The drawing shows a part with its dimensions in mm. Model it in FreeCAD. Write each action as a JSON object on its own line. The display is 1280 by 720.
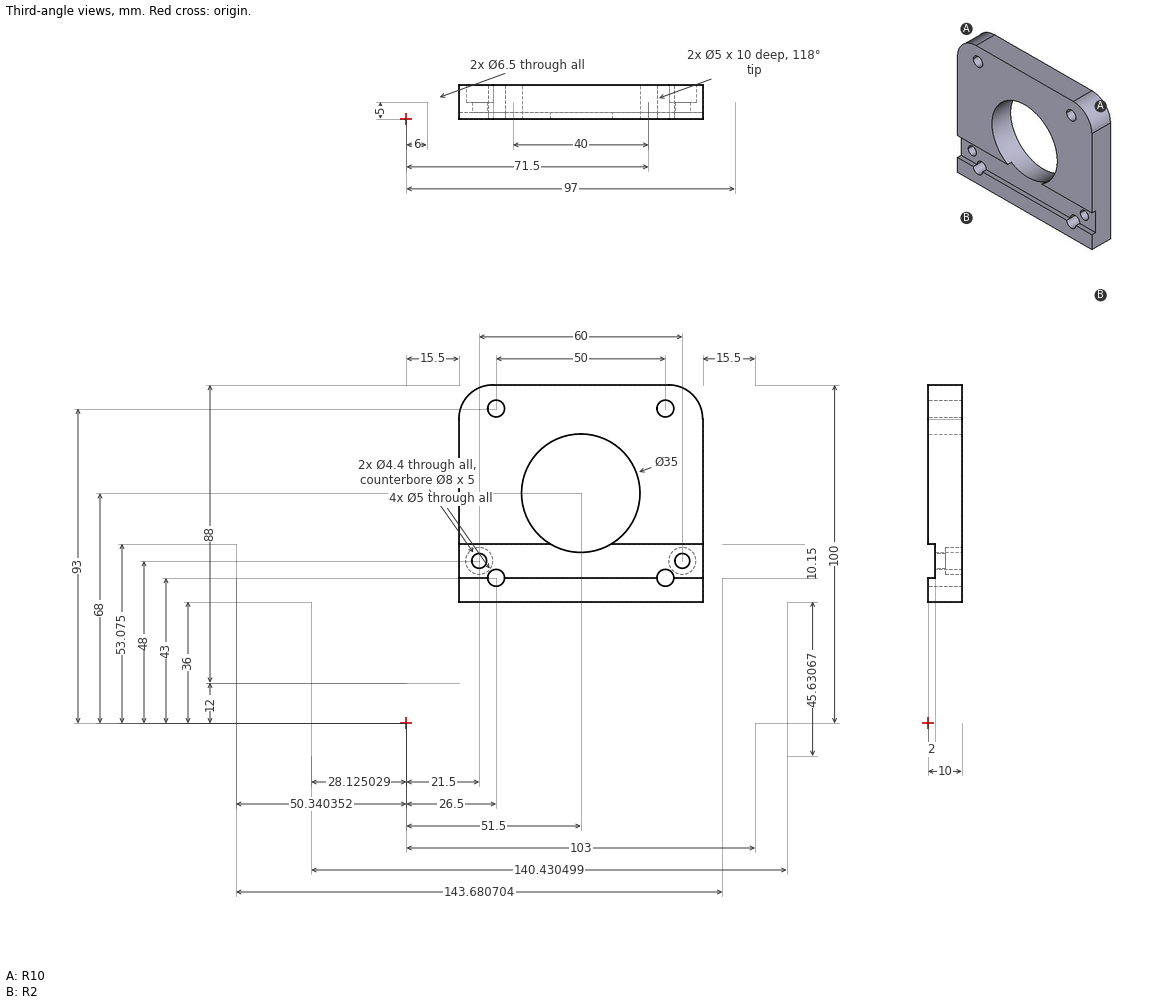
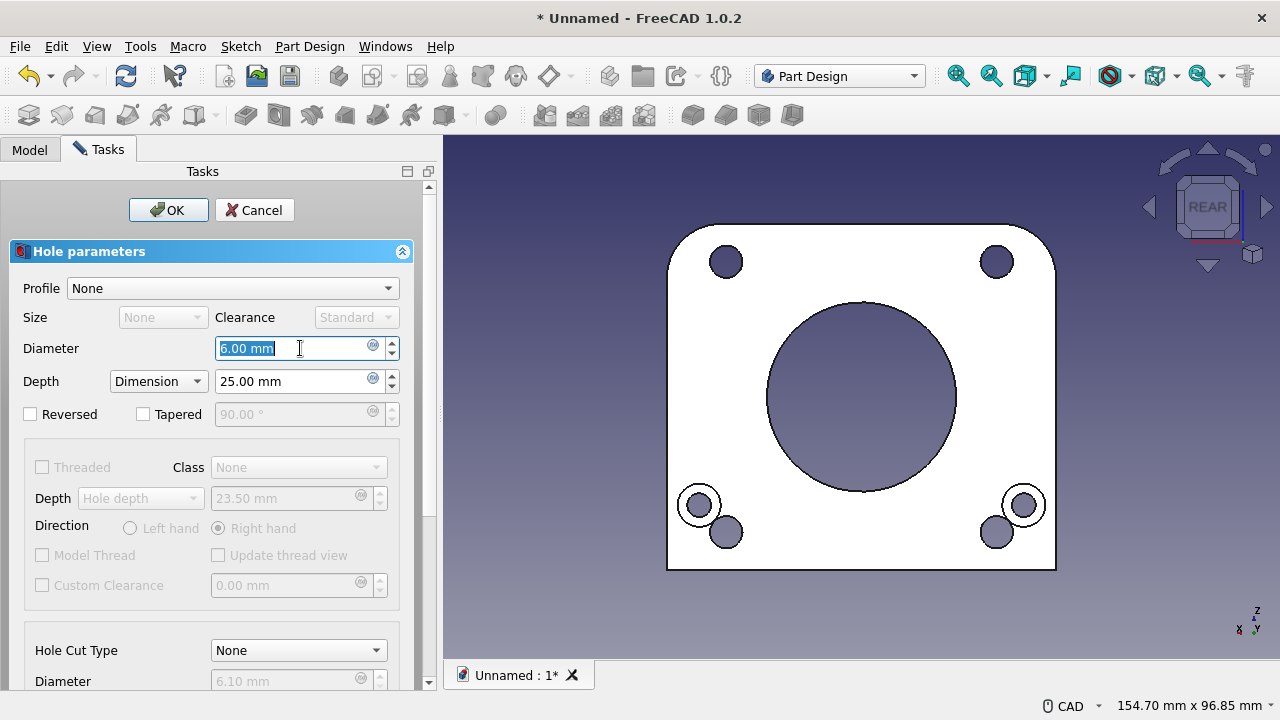
{"action": "type", "text": "5"}
{"action": "key", "text": "Tab"}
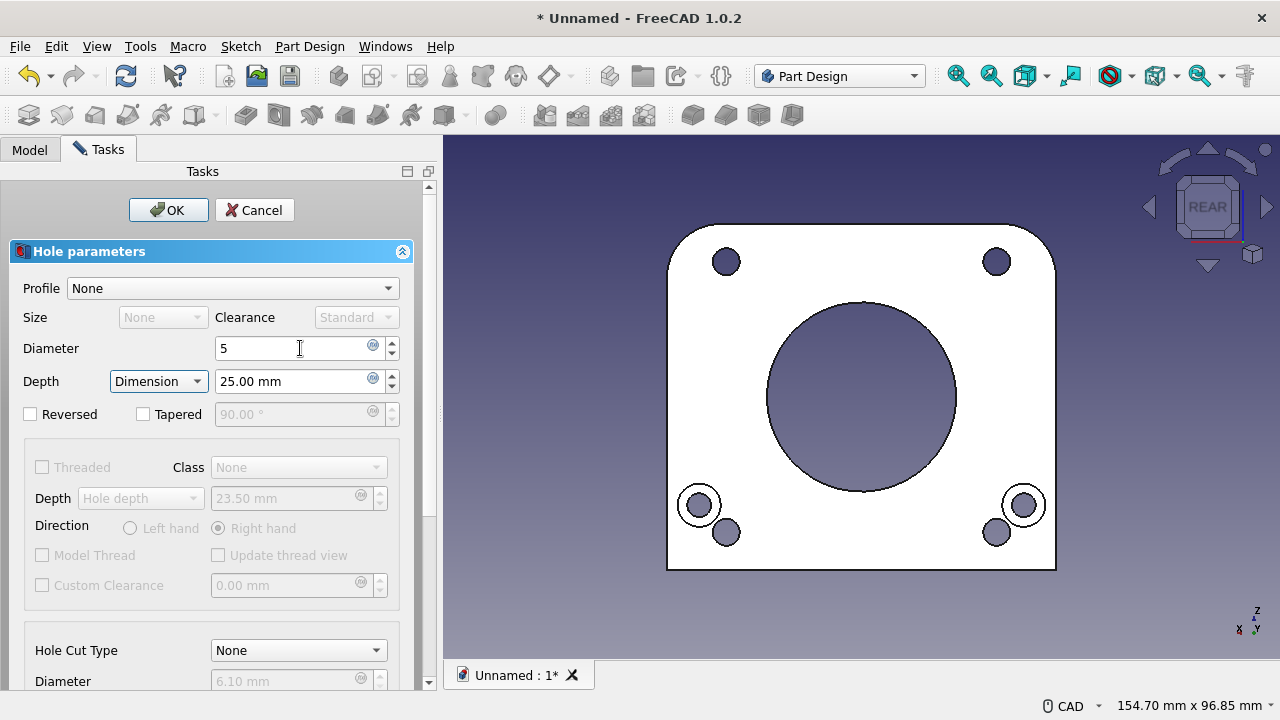
{"action": "left_click", "coordinate": [160, 382]}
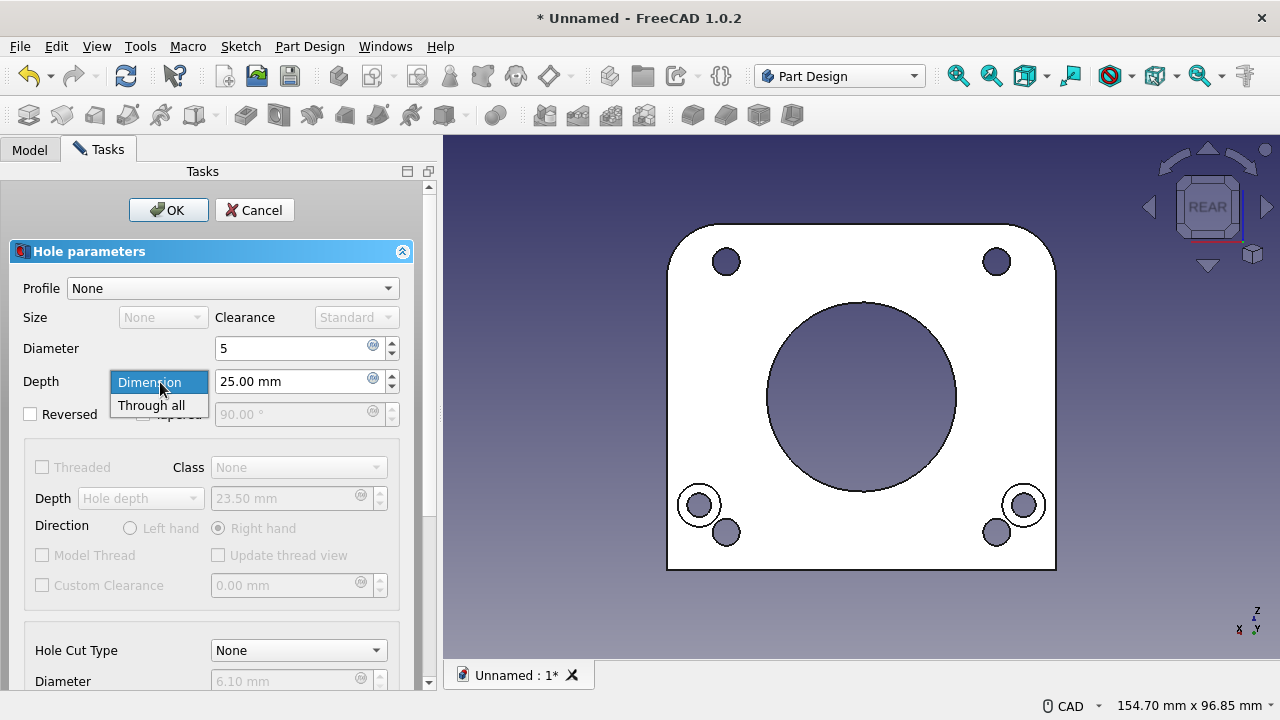
{"action": "left_click", "coordinate": [158, 406]}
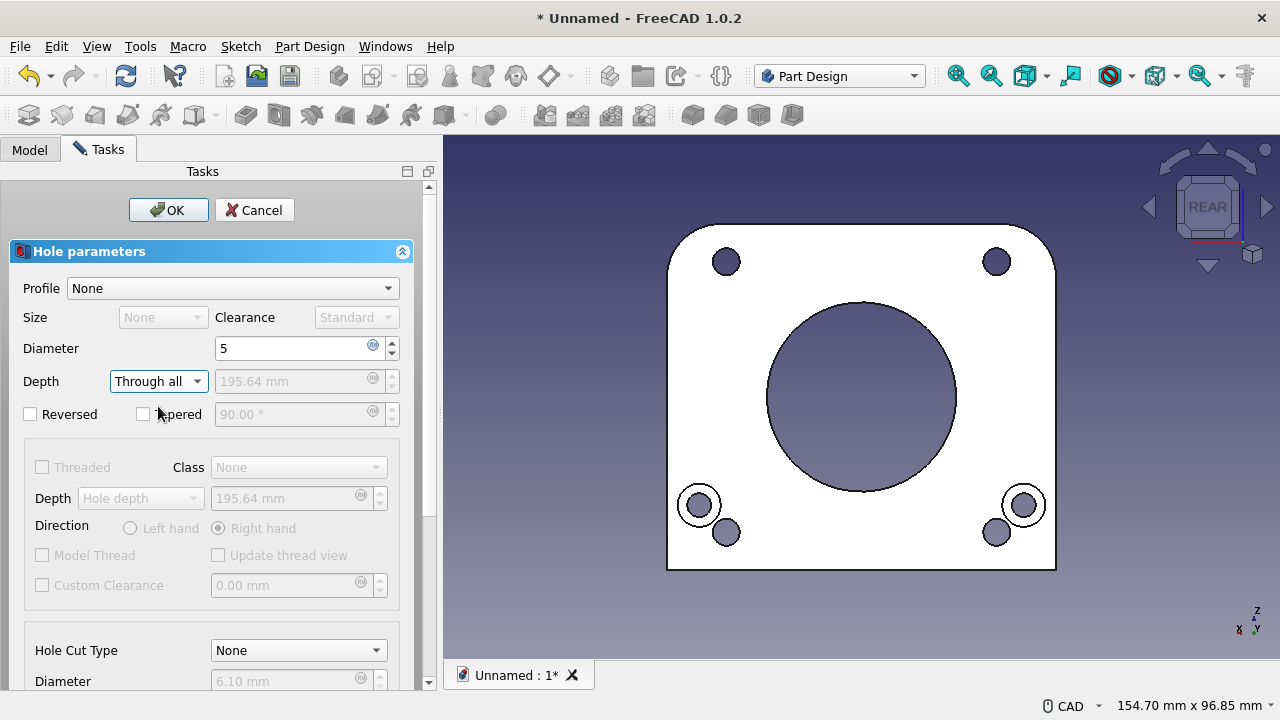
{"action": "left_click", "coordinate": [169, 210]}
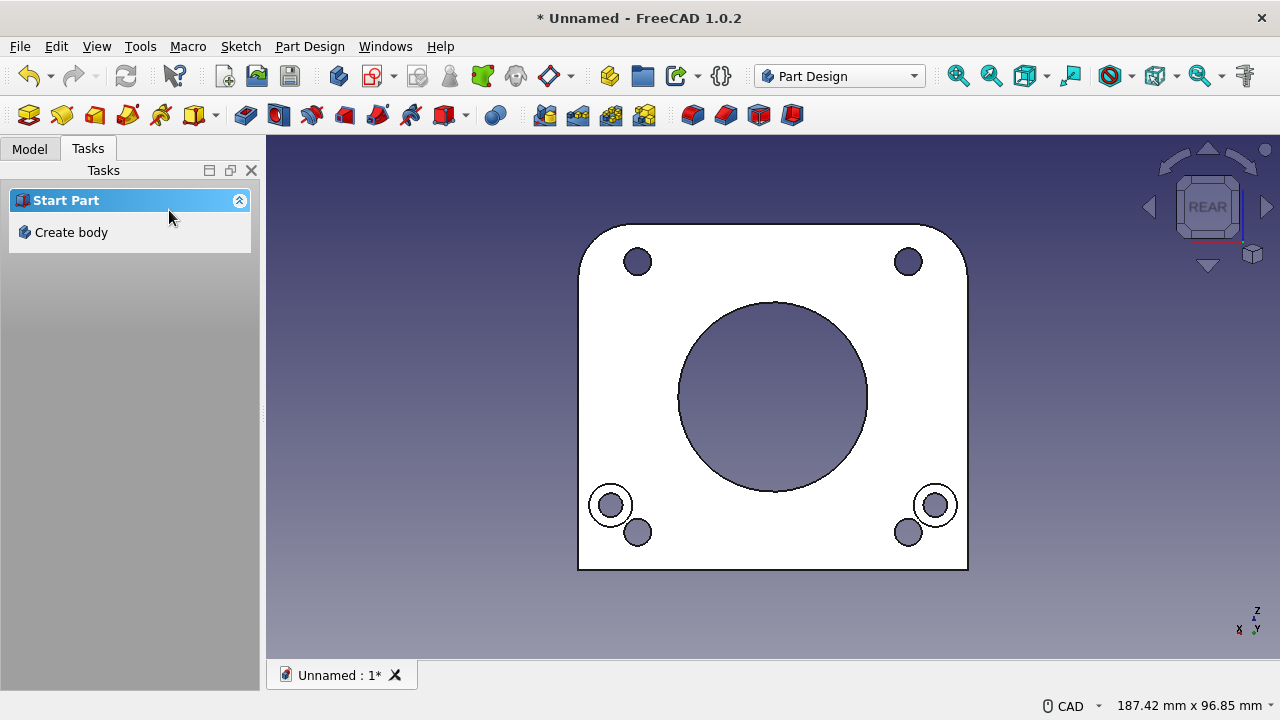
{"action": "key", "text": "0"}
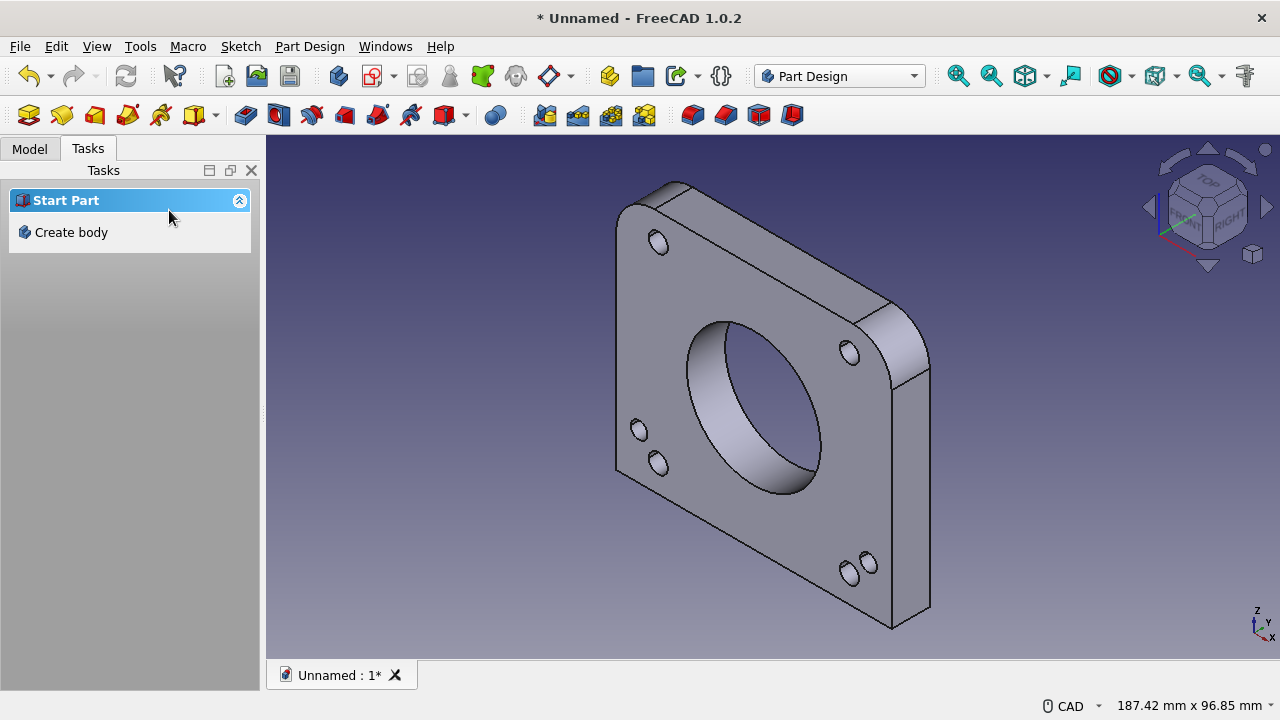
{"action": "left_click", "coordinate": [675, 442]}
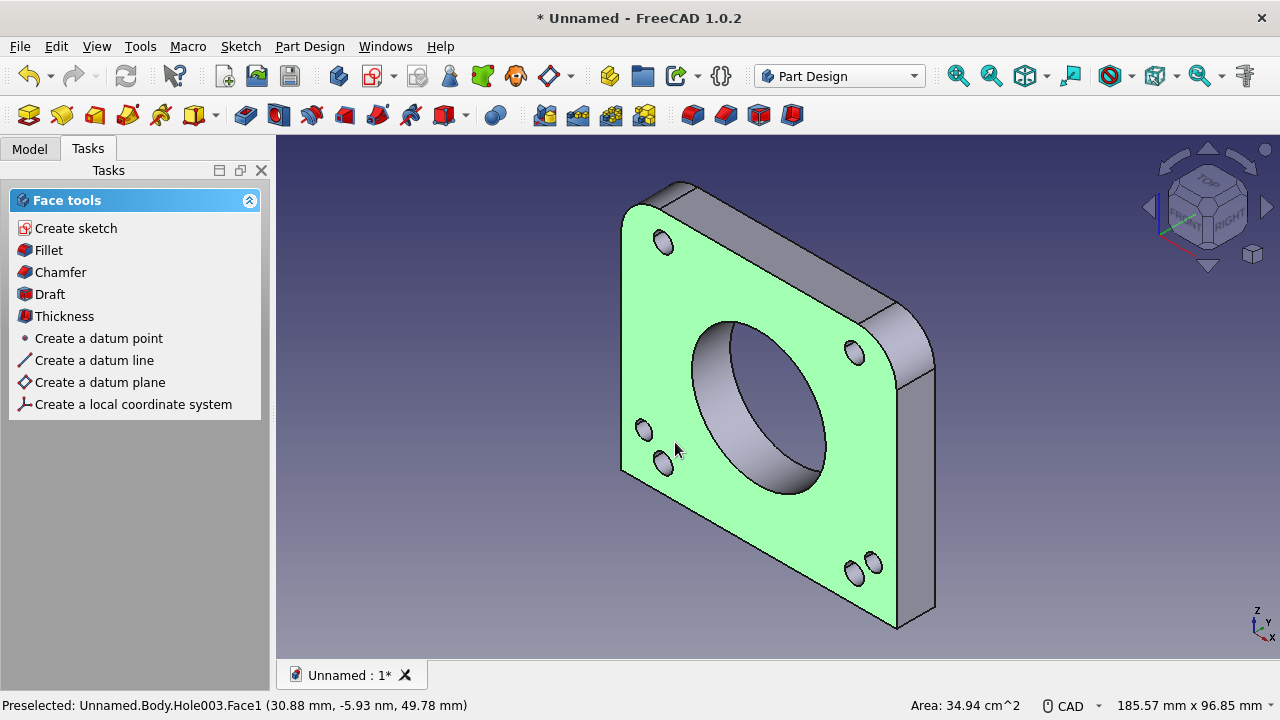
{"action": "left_click", "coordinate": [372, 76]}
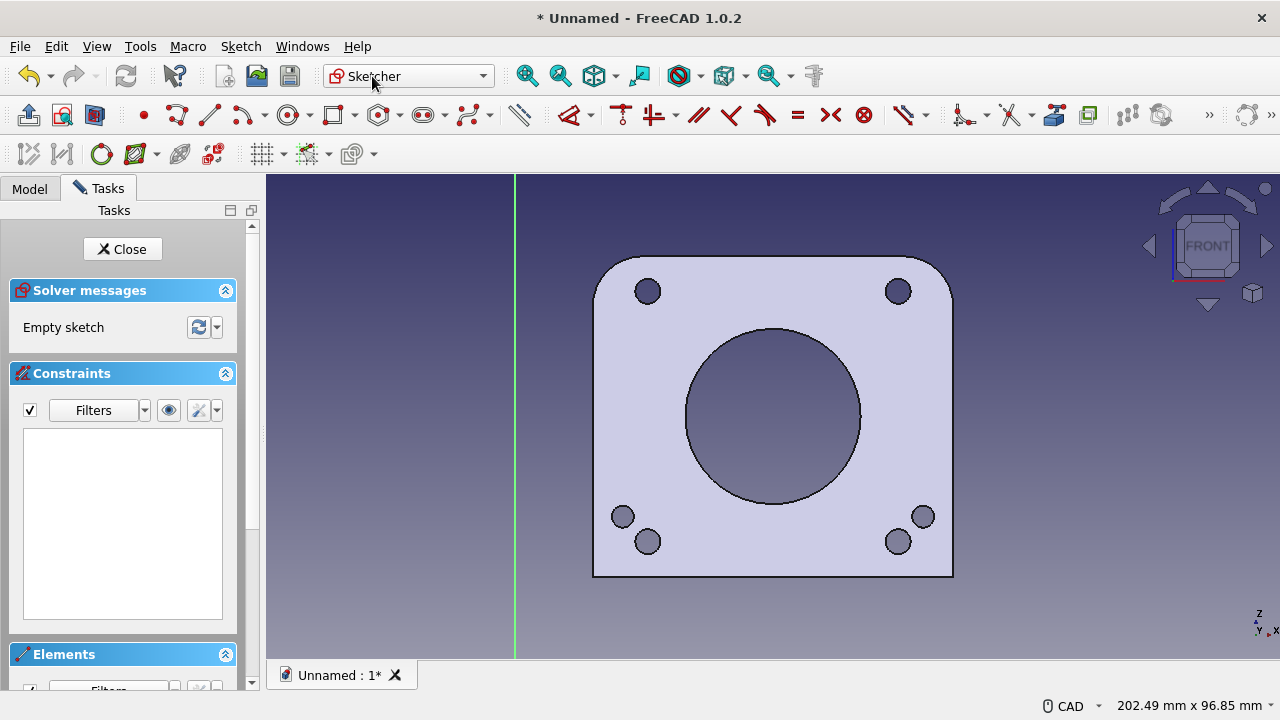
{"action": "scroll", "coordinate": [871, 202], "scroll_direction": "down", "scroll_amount": 2}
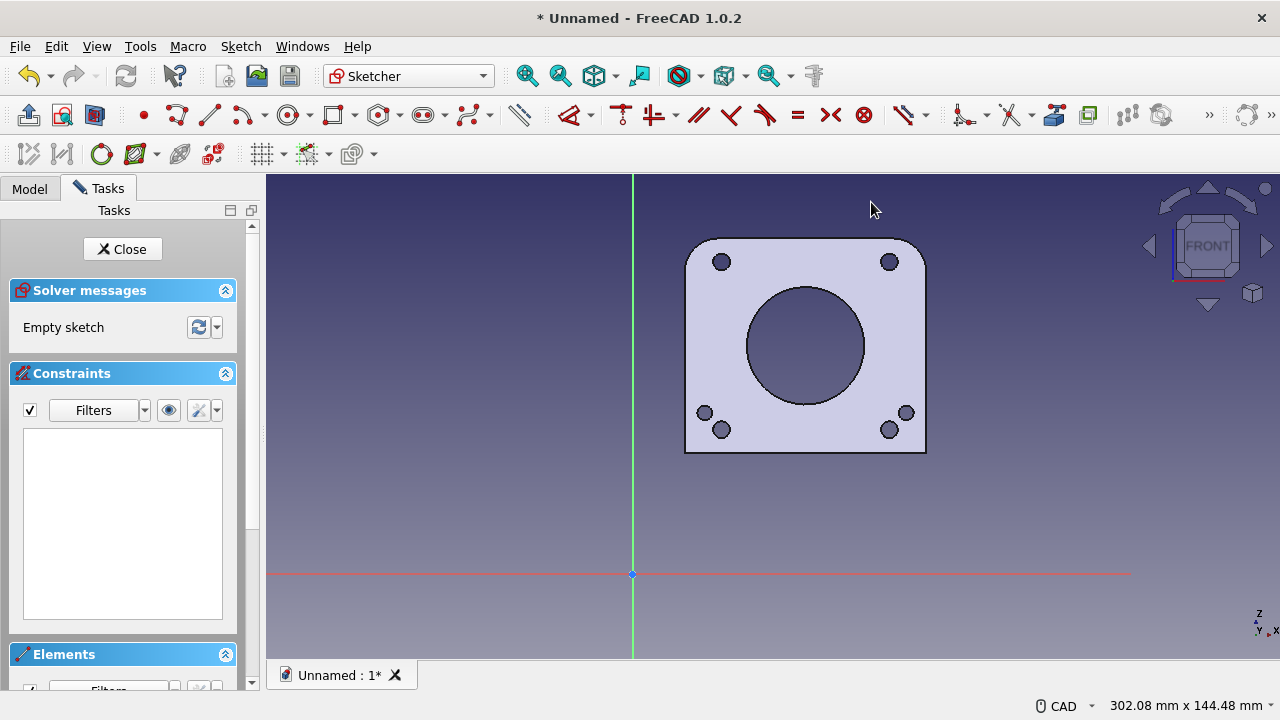
{"action": "left_click", "coordinate": [332, 116]}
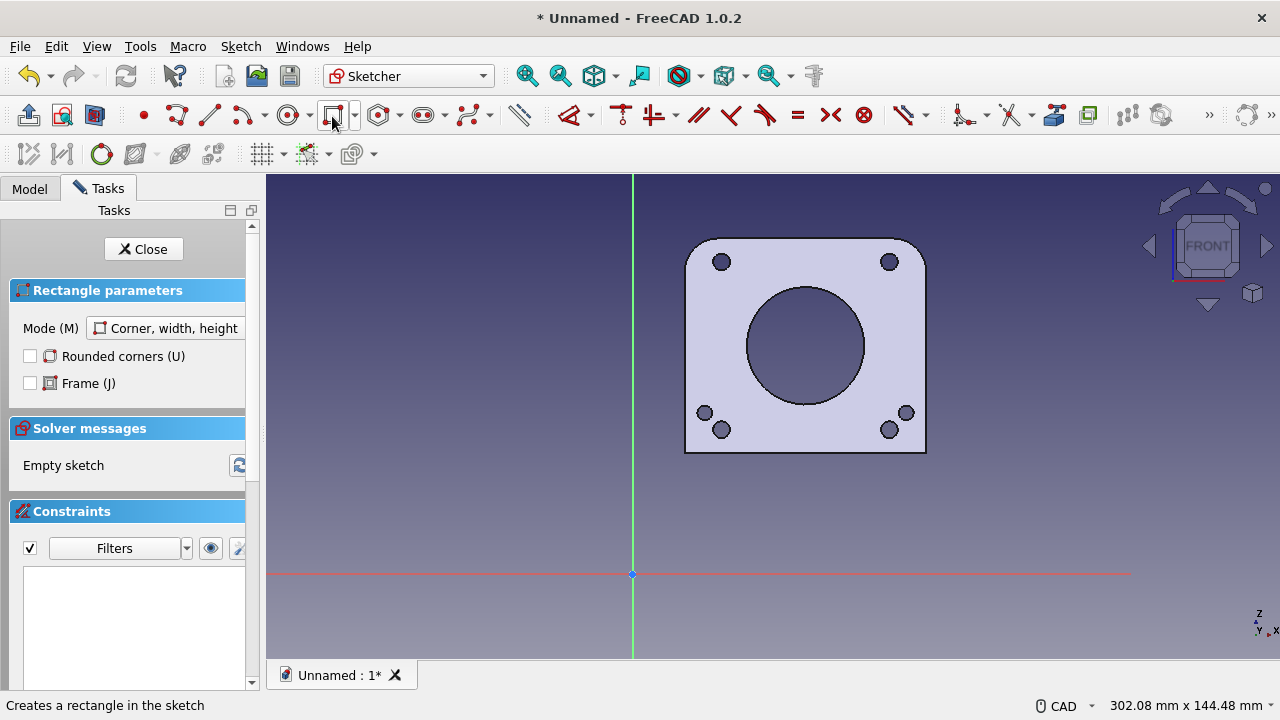
{"action": "left_click", "coordinate": [464, 396]}
{"action": "mouse_move", "coordinate": [946, 430]}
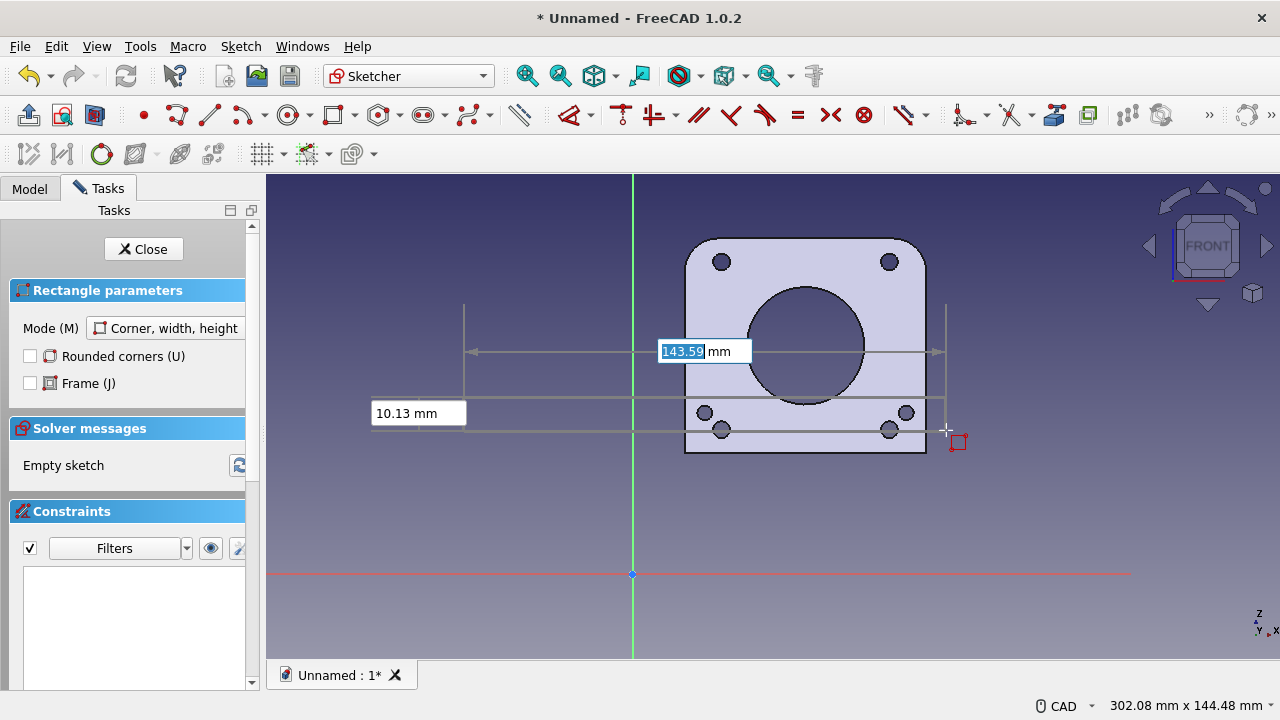
{"action": "type", "text": "143.680704"}
{"action": "key", "text": "Tab"}
{"action": "type", "text": "10.15"}
{"action": "key", "text": "Return"}
{"action": "key", "text": "Escape"}